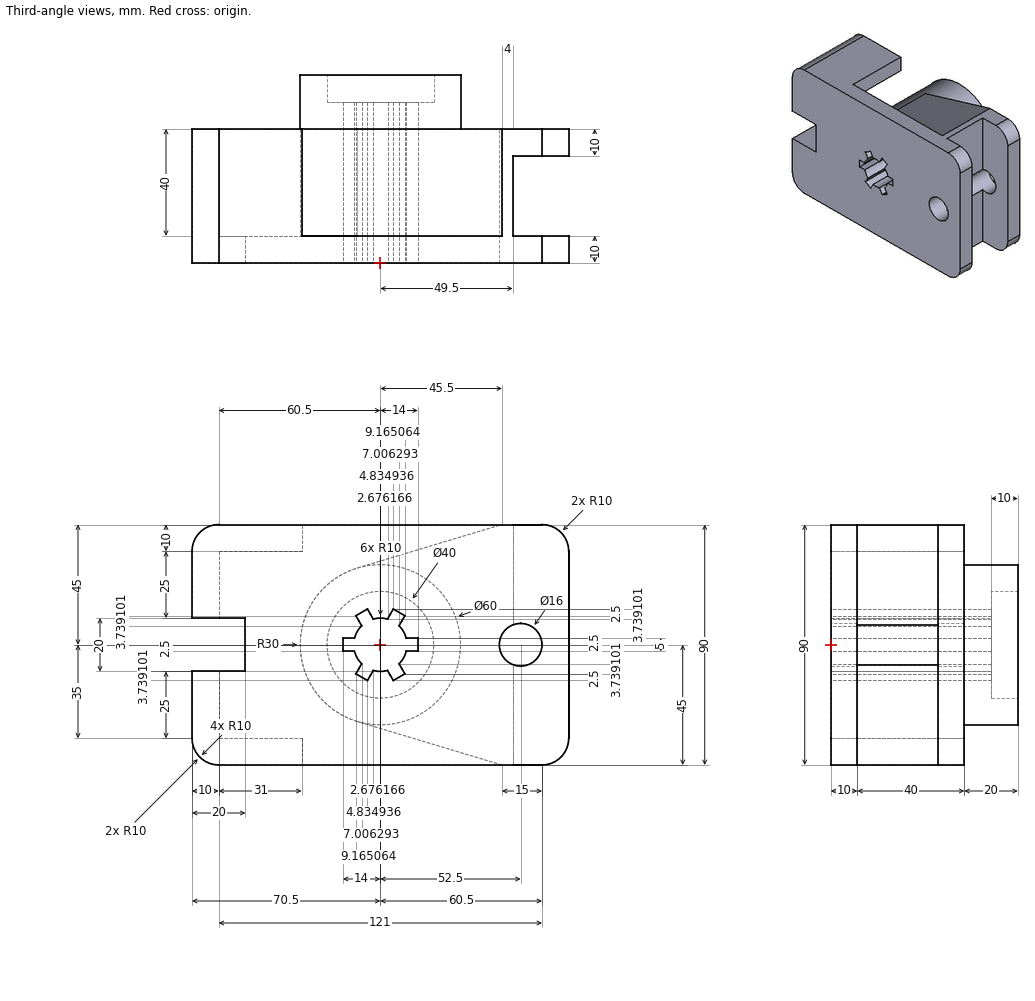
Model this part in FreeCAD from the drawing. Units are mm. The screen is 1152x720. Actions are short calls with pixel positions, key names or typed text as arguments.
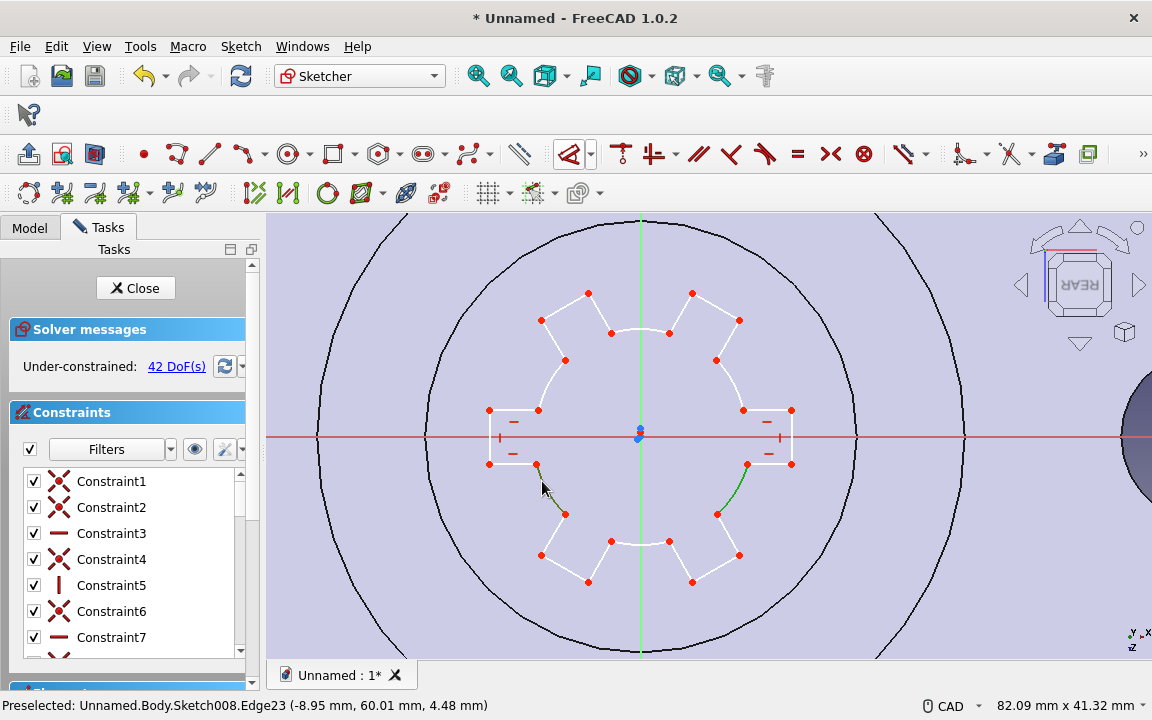
click(621, 154)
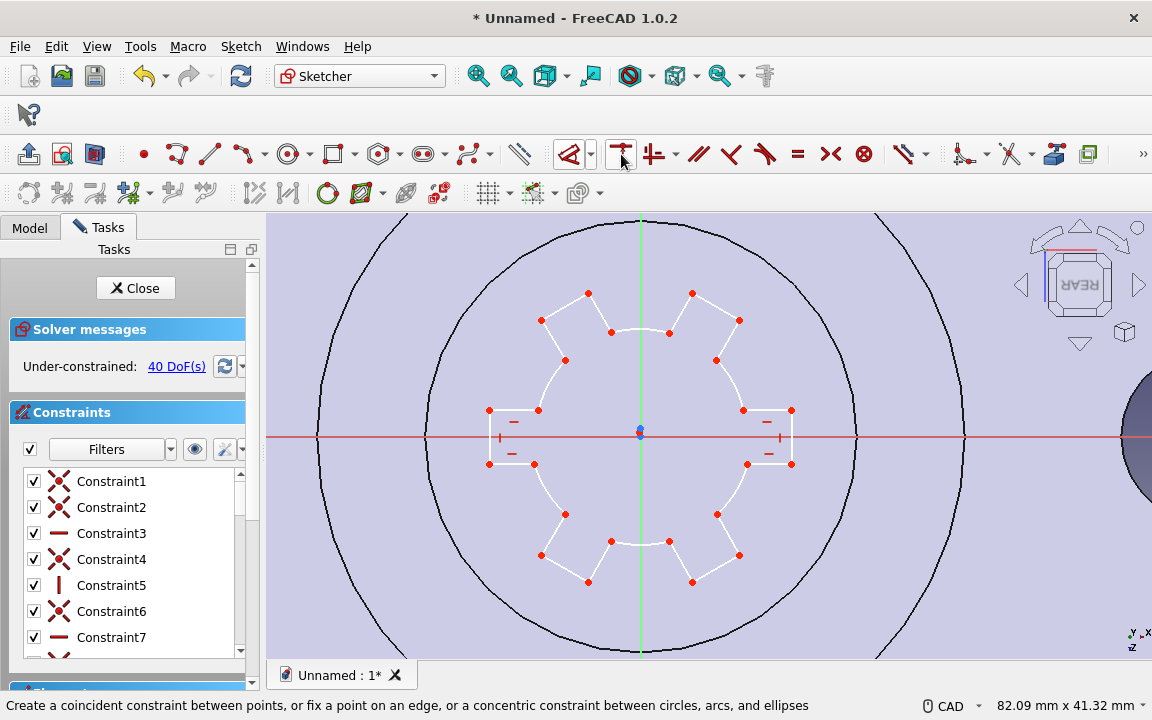
click(729, 501)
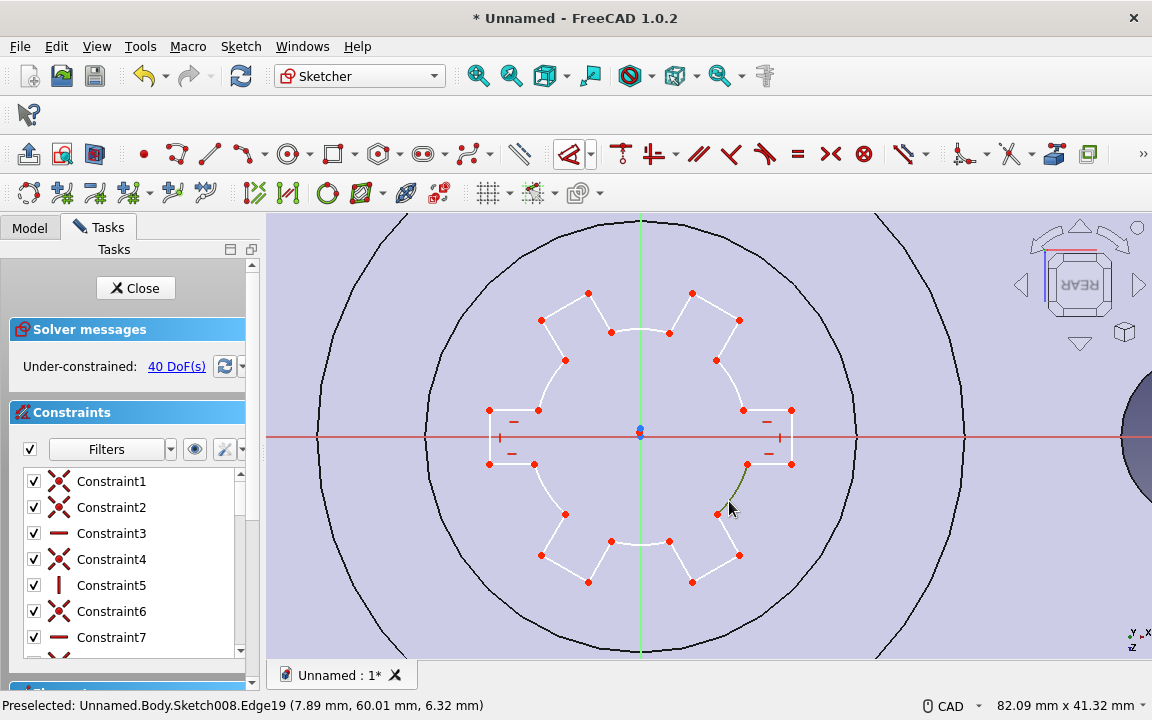
click(629, 544)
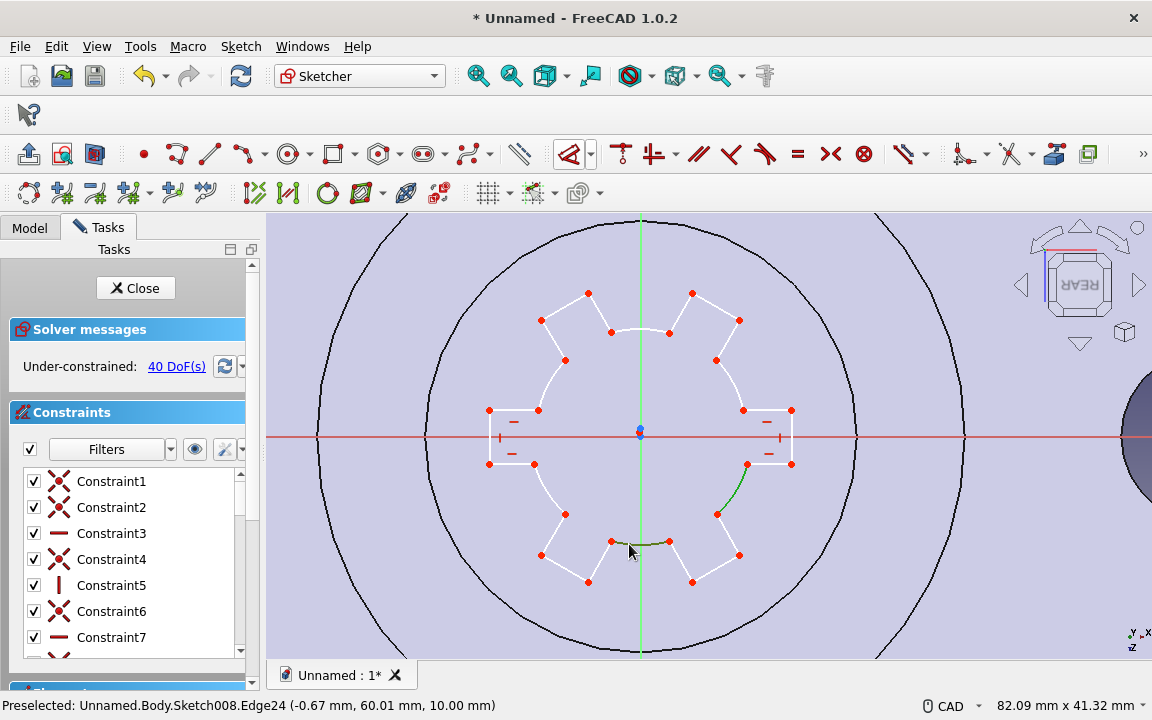
click(621, 154)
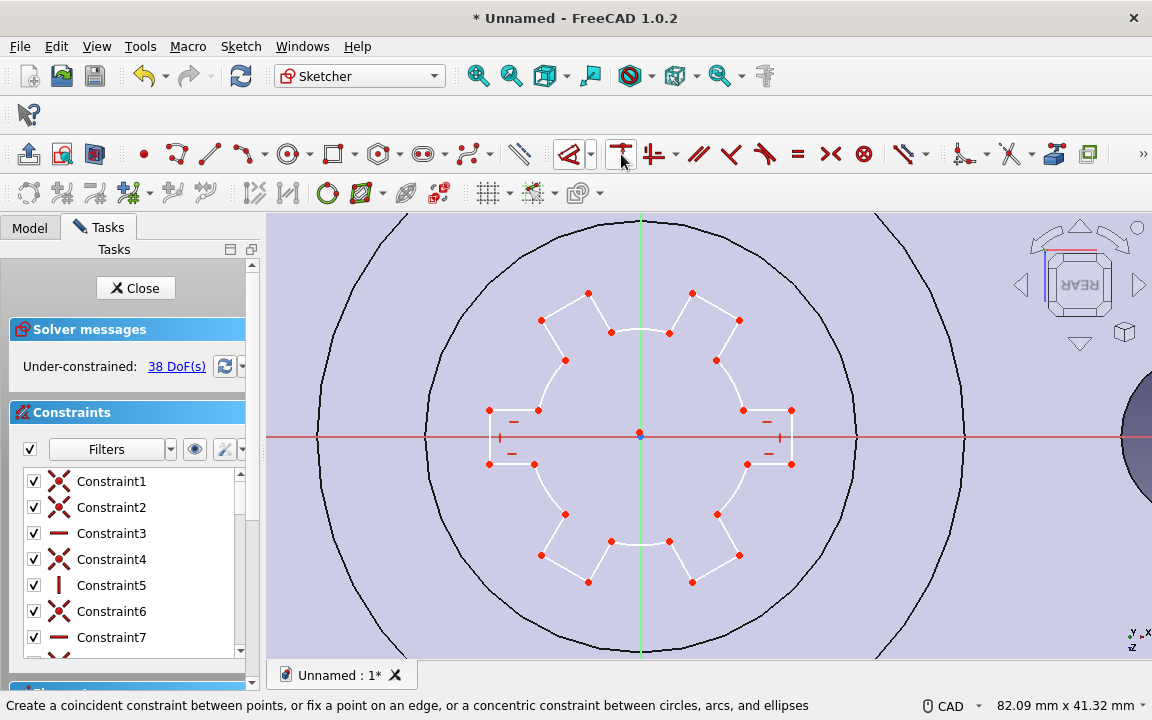
drag(630, 423, 651, 447)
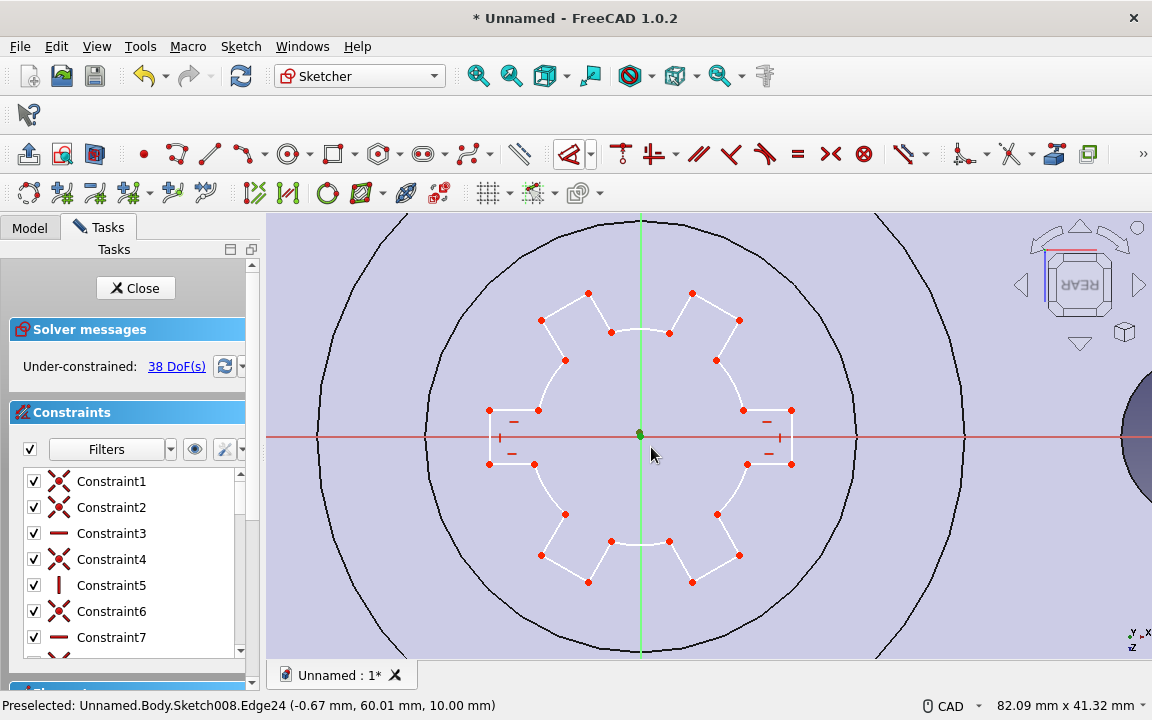
click(621, 154)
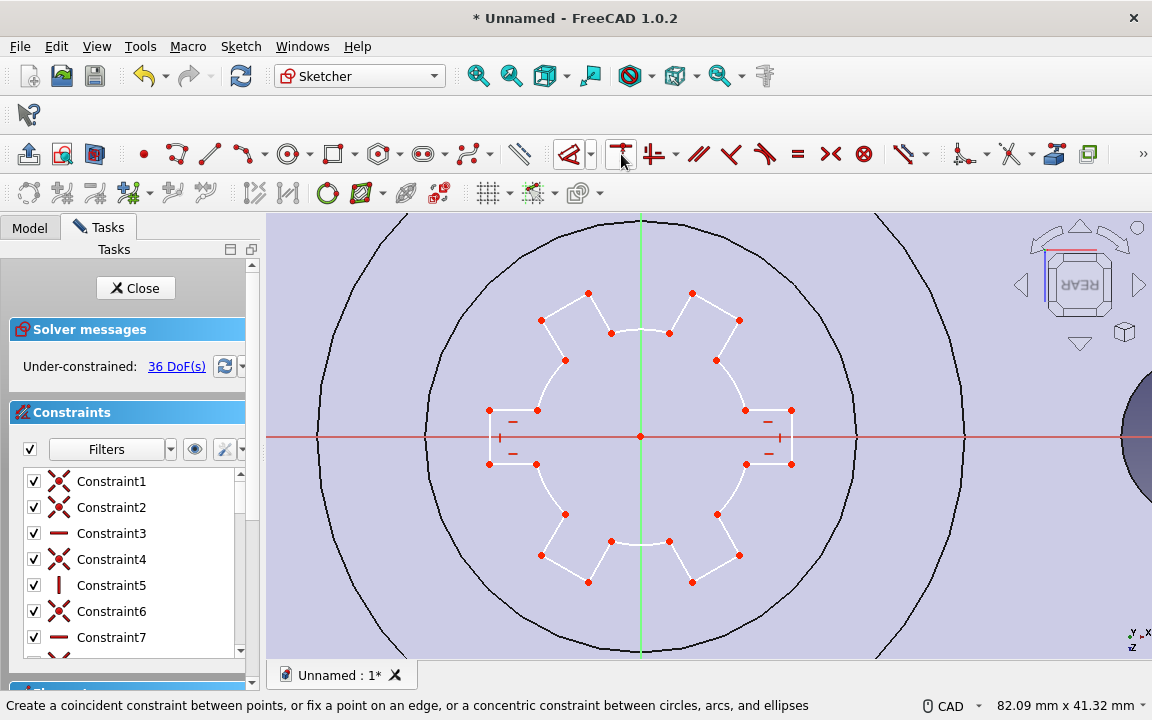
click(729, 501)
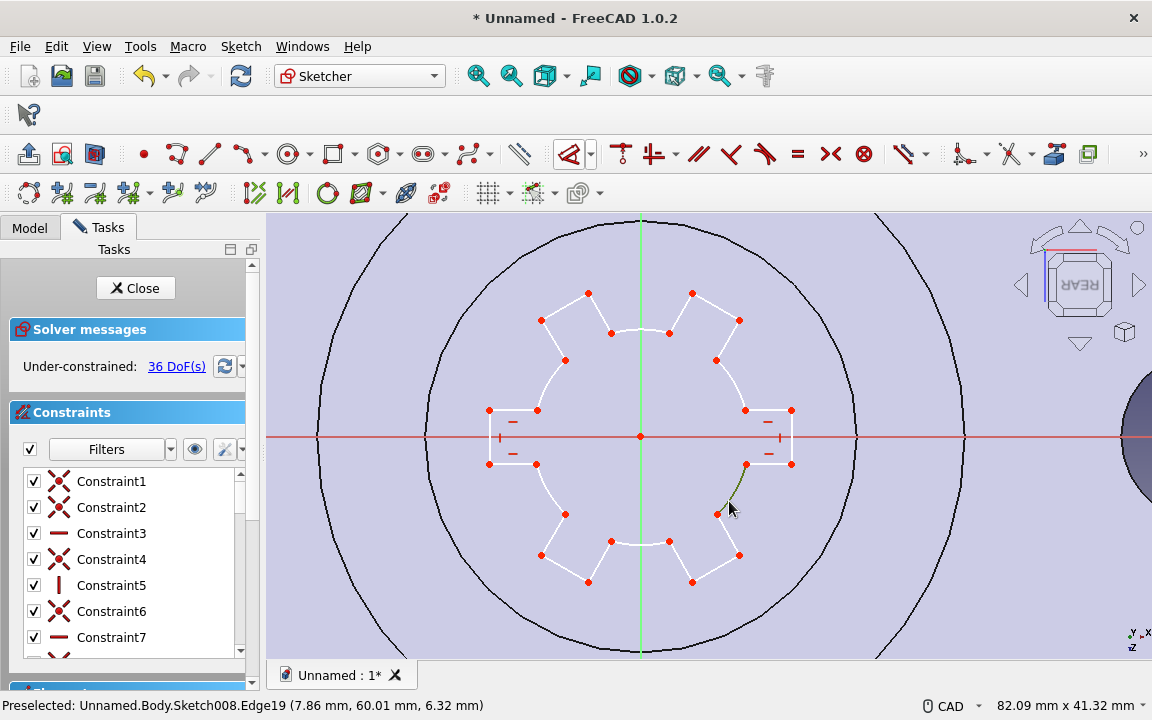
click(740, 394)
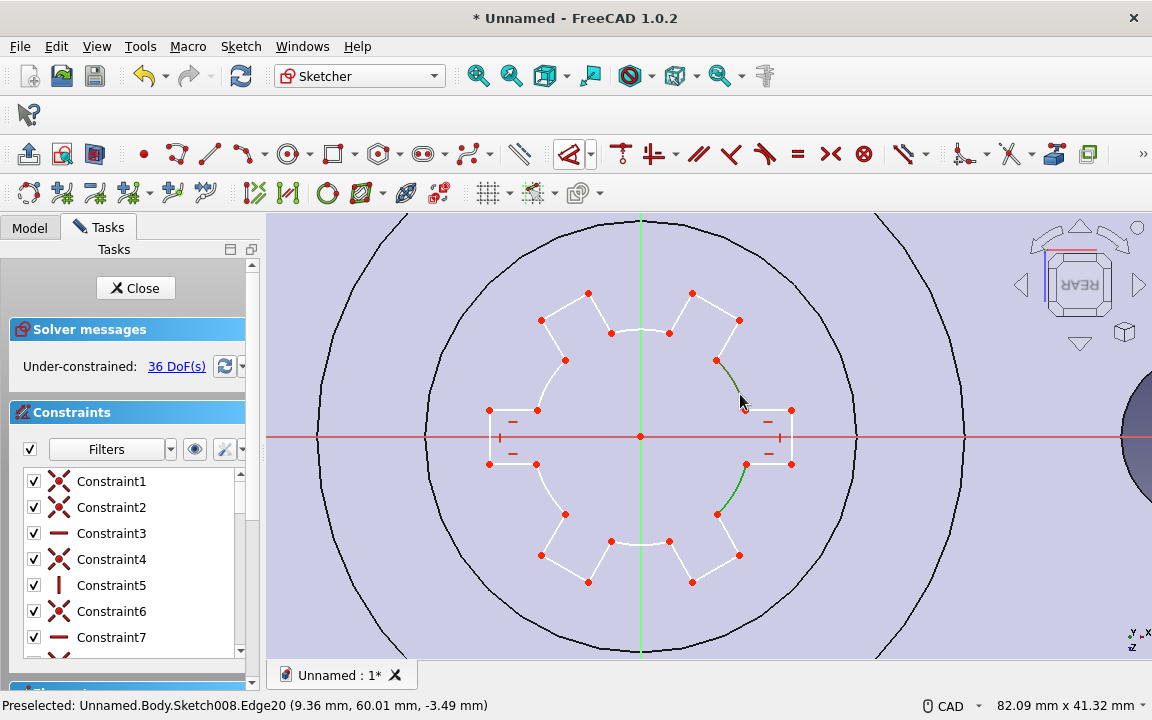
click(652, 330)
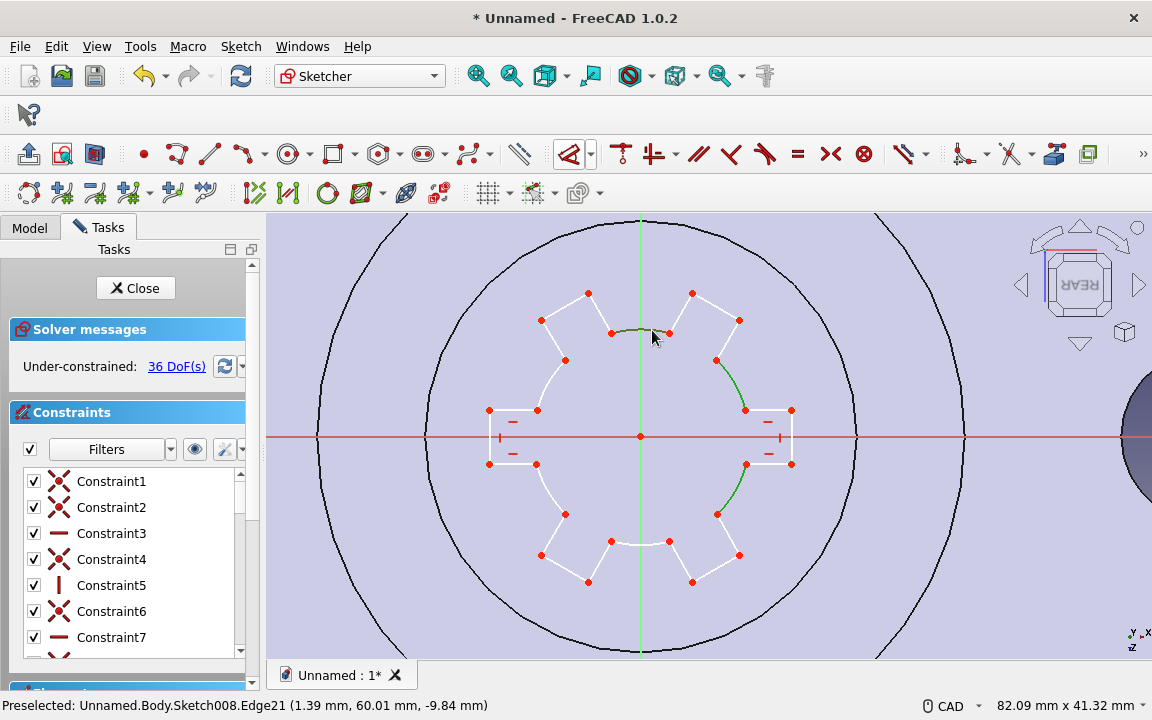
click(555, 374)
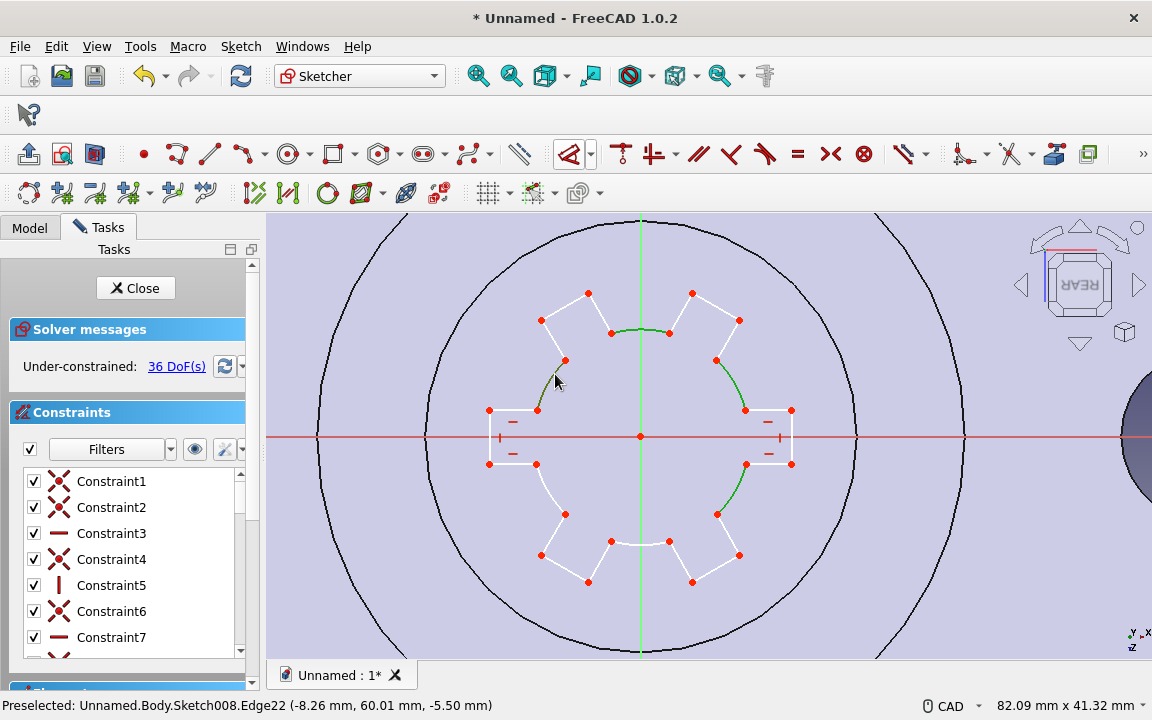
click(543, 481)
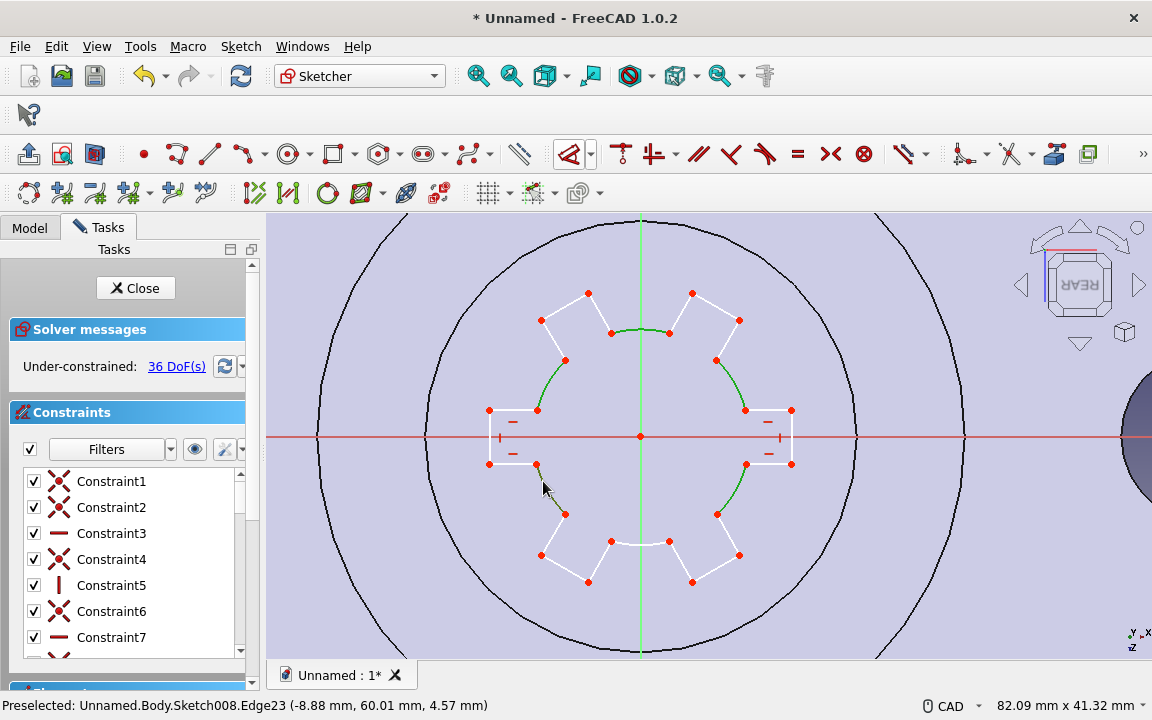
click(629, 545)